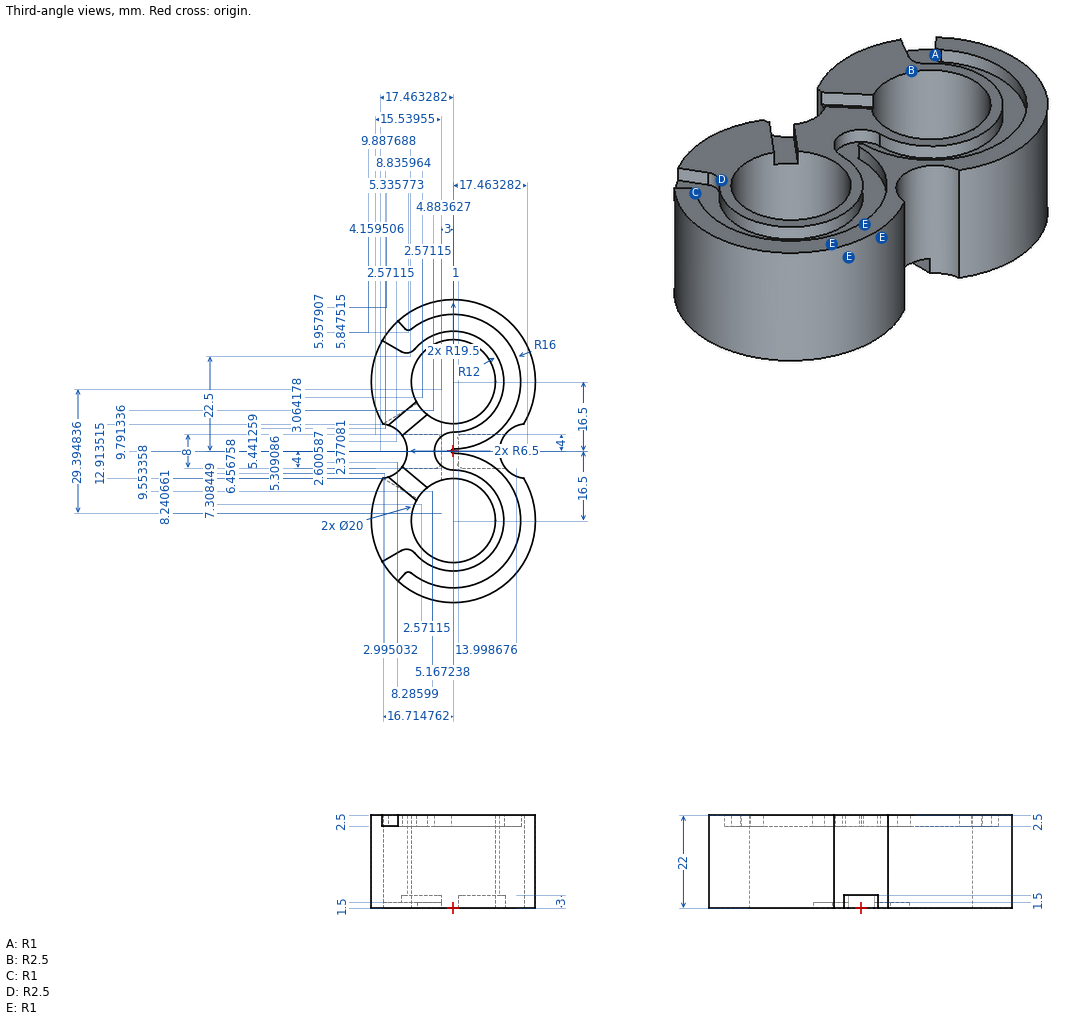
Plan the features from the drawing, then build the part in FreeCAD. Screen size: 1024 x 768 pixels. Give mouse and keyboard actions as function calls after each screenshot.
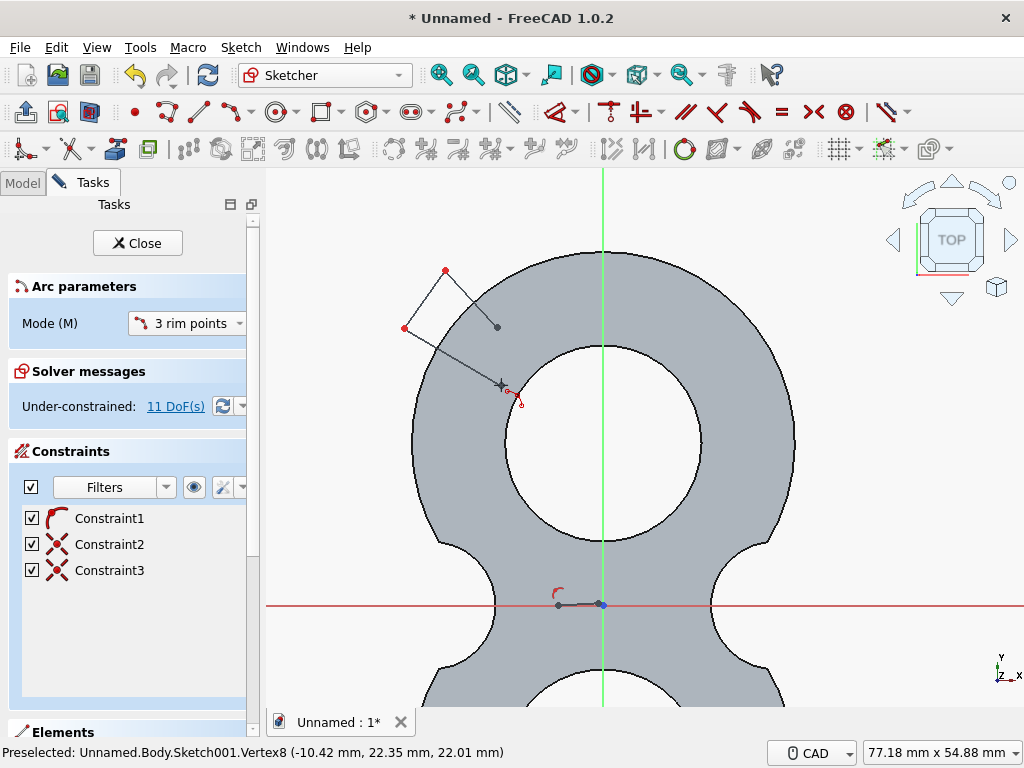
scroll(598, 606, up, 6)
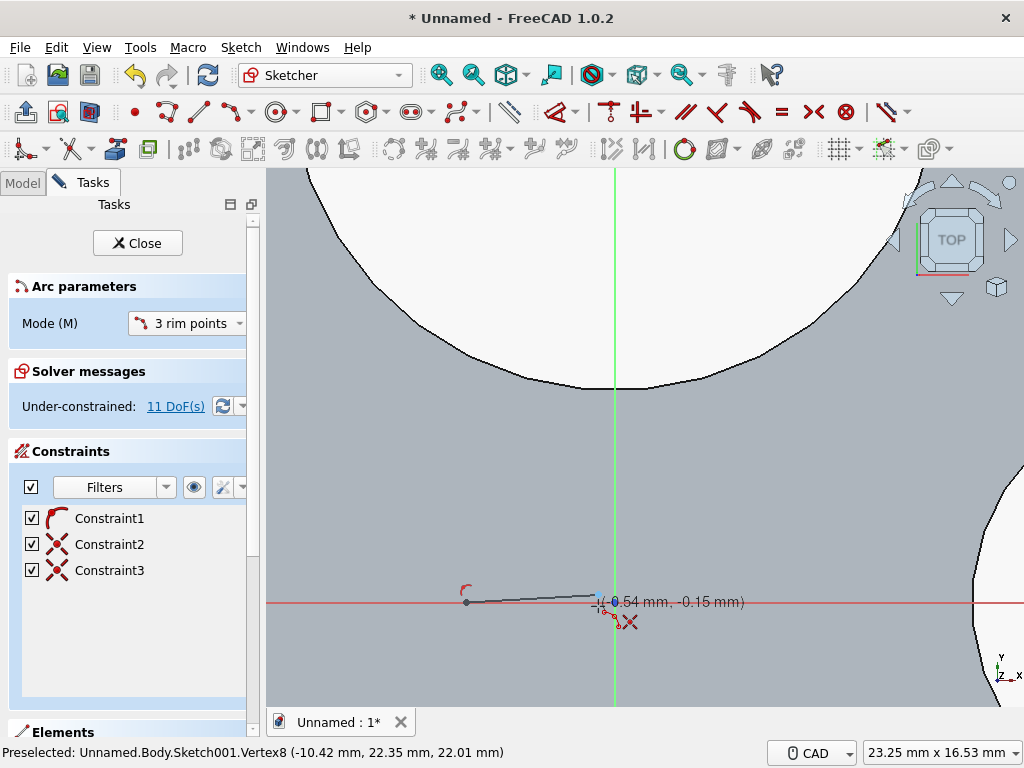
click(598, 595)
click(615, 586)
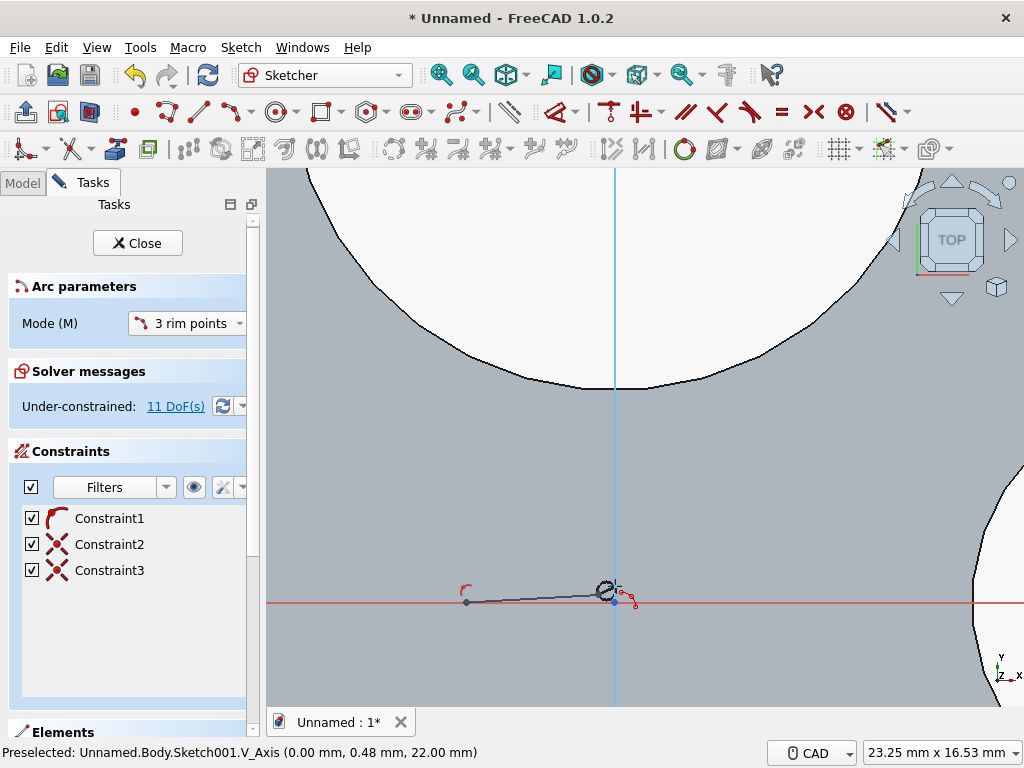
scroll(603, 591, up, 7)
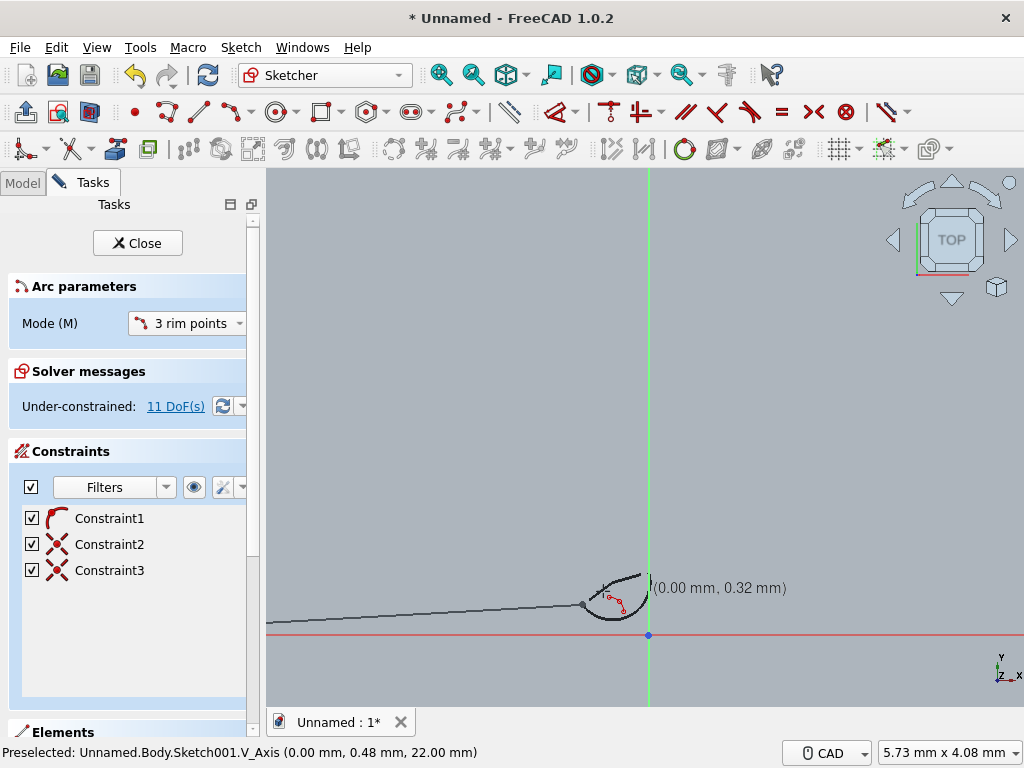
click(602, 589)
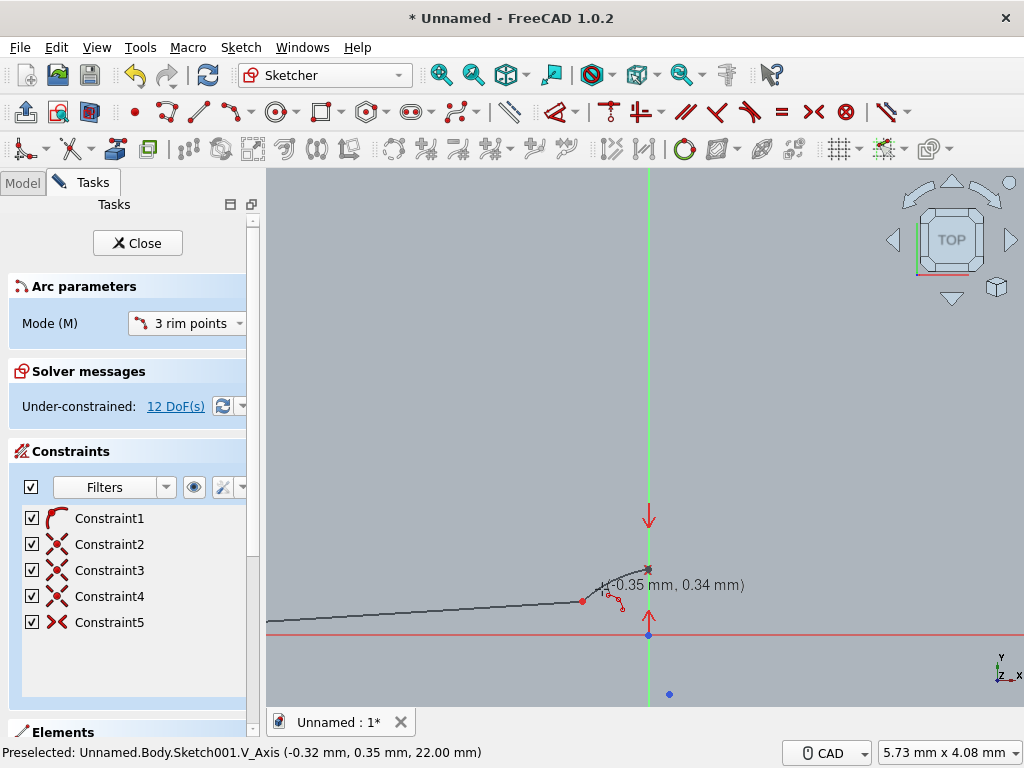
scroll(599, 603, down, 13)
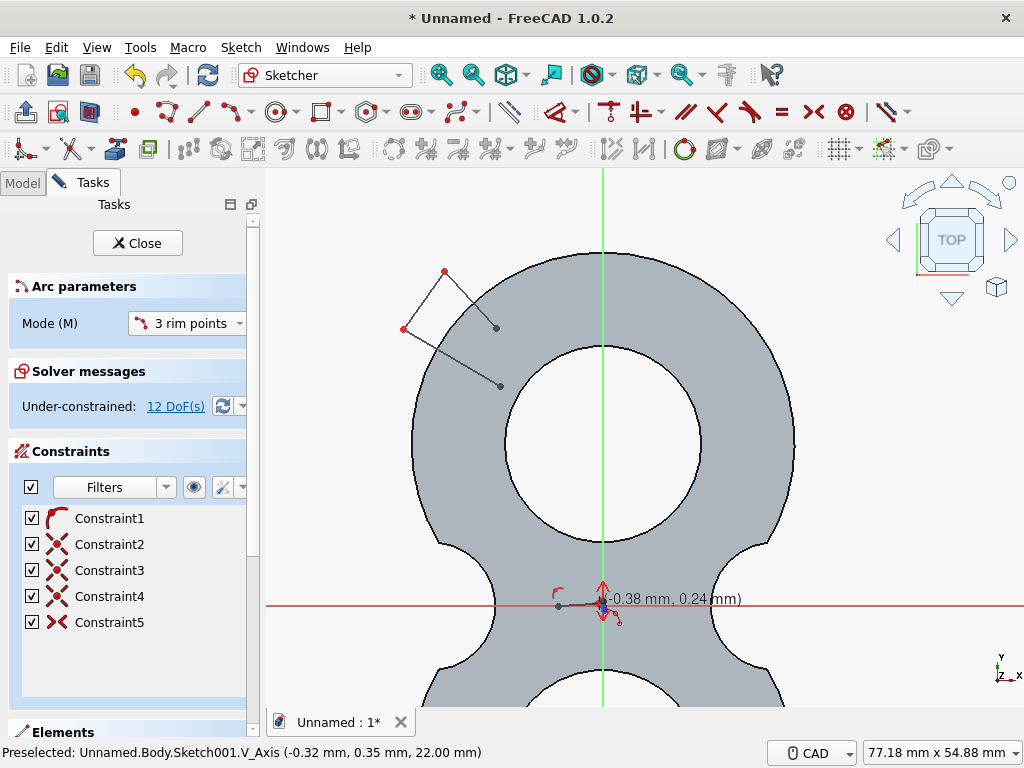
scroll(603, 601, up, 6)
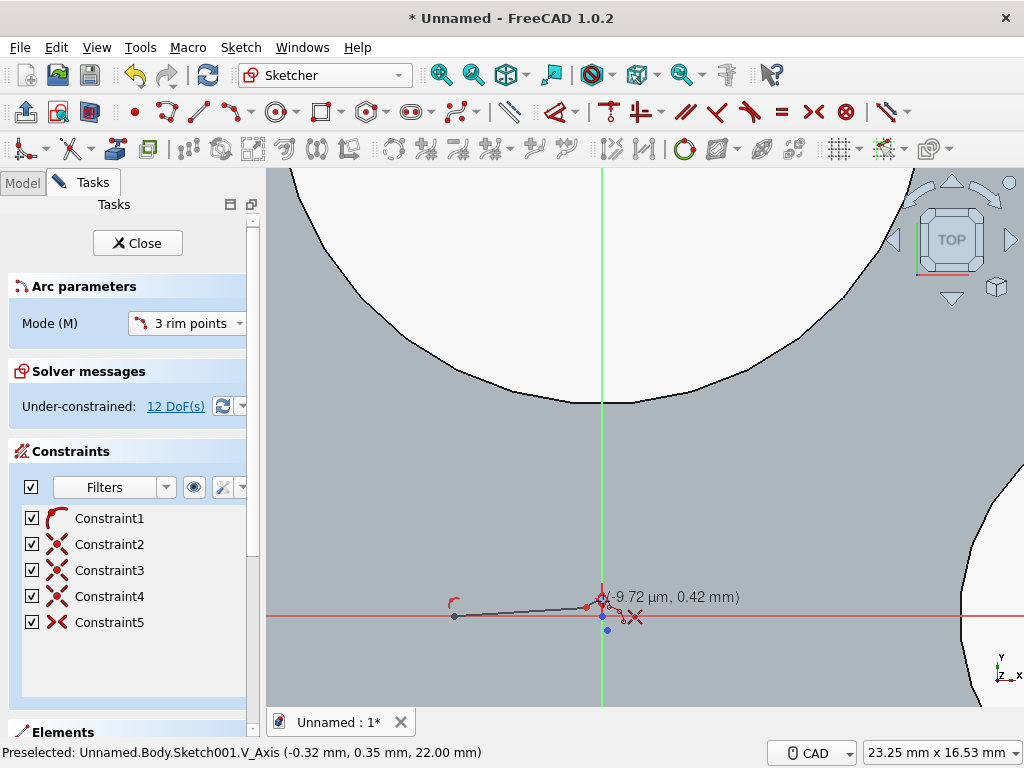
click(602, 600)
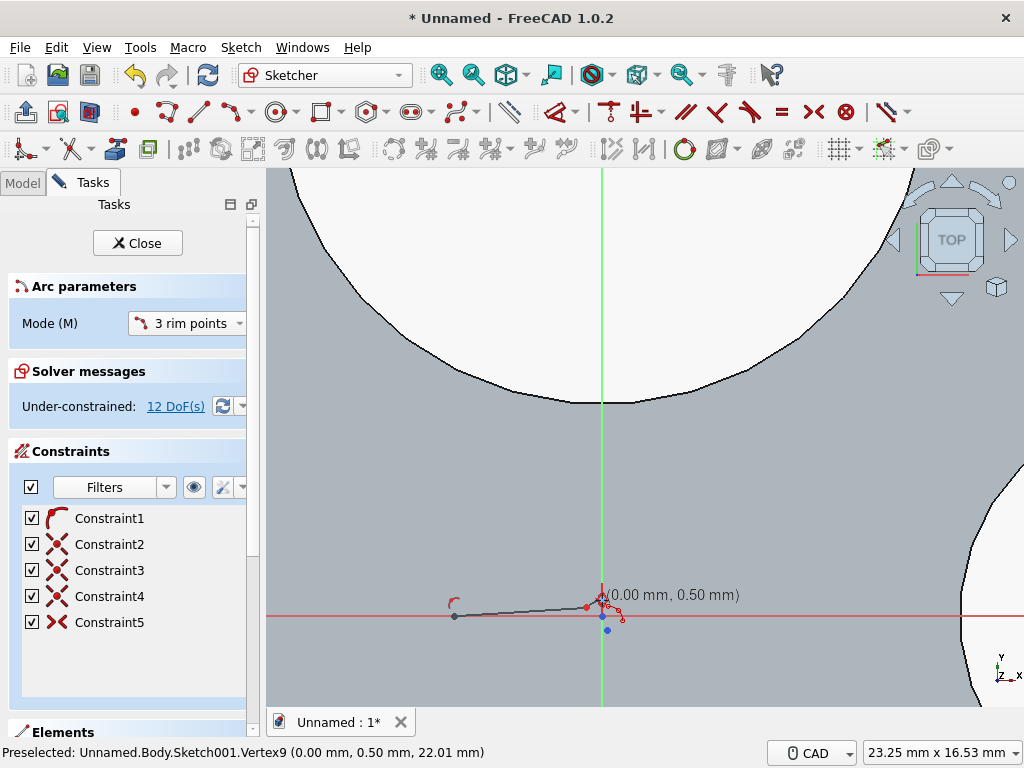
scroll(603, 601, down, 6)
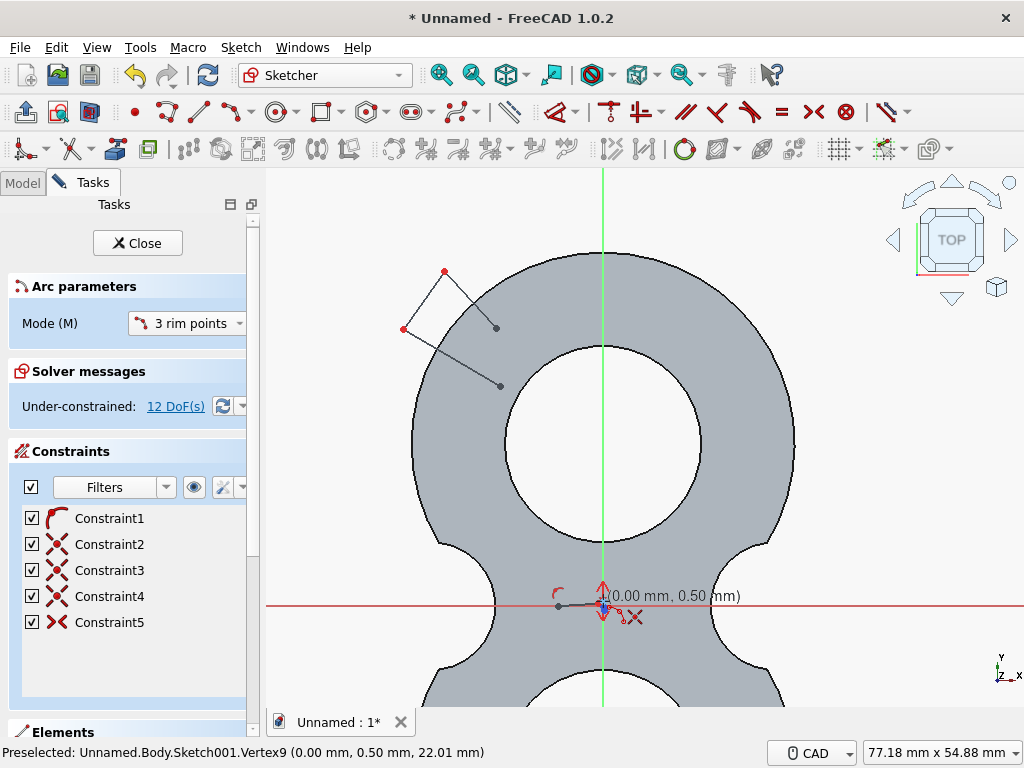
click(497, 329)
click(750, 387)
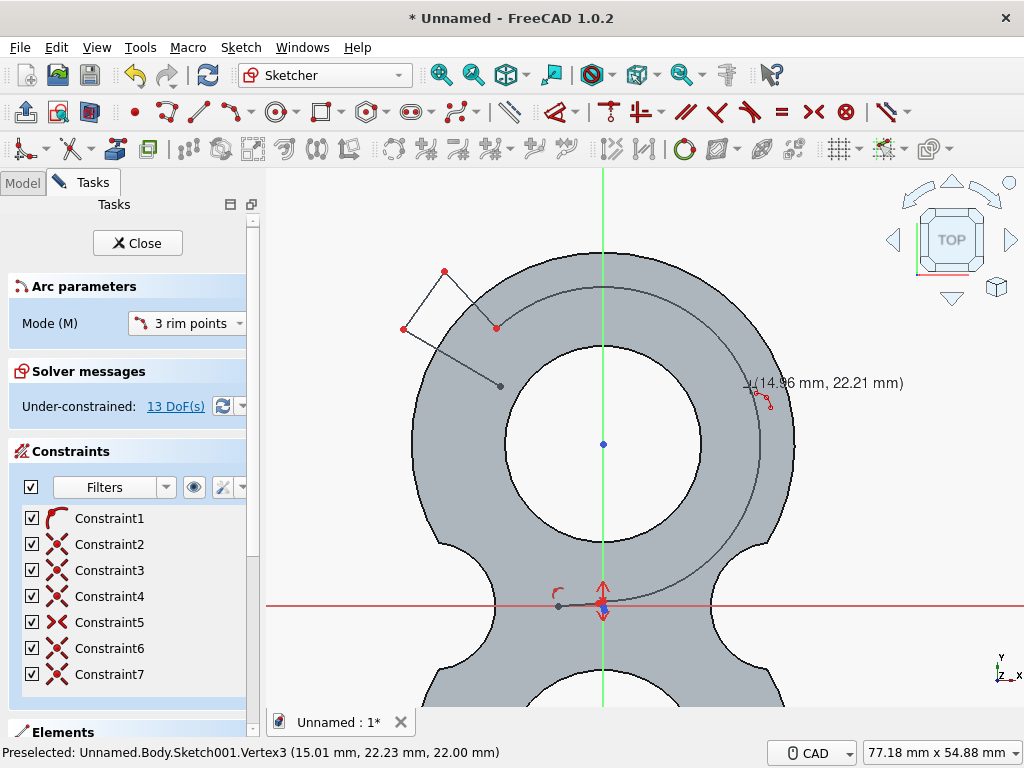
click(501, 387)
click(603, 562)
click(705, 385)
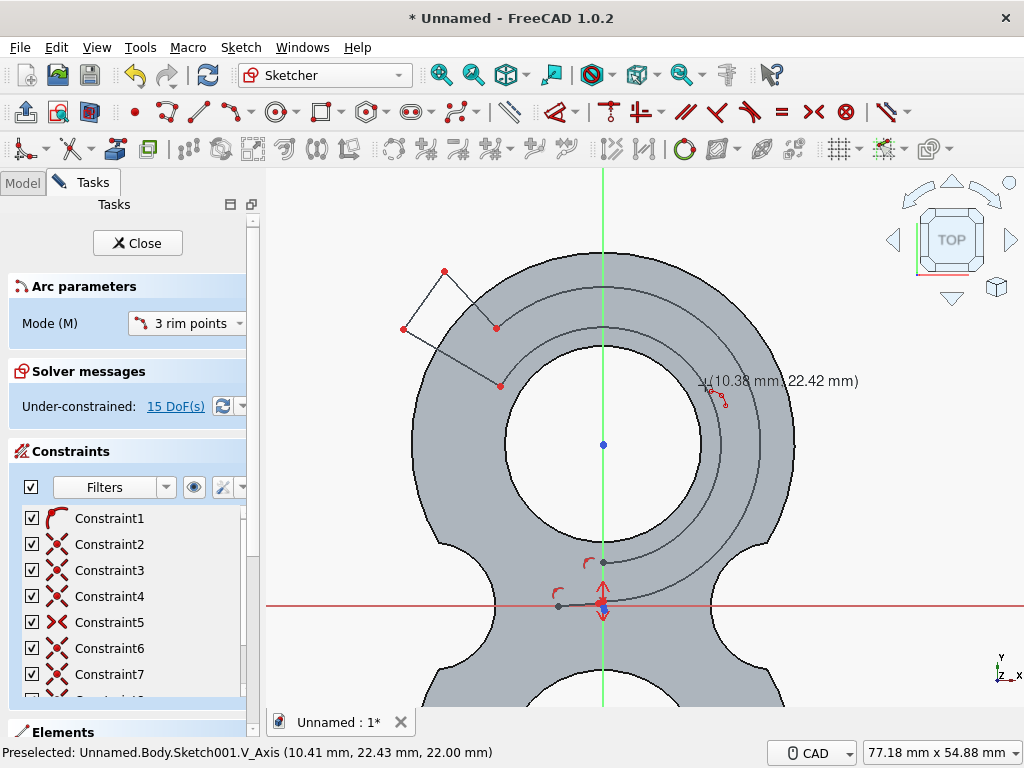
click(603, 563)
click(558, 606)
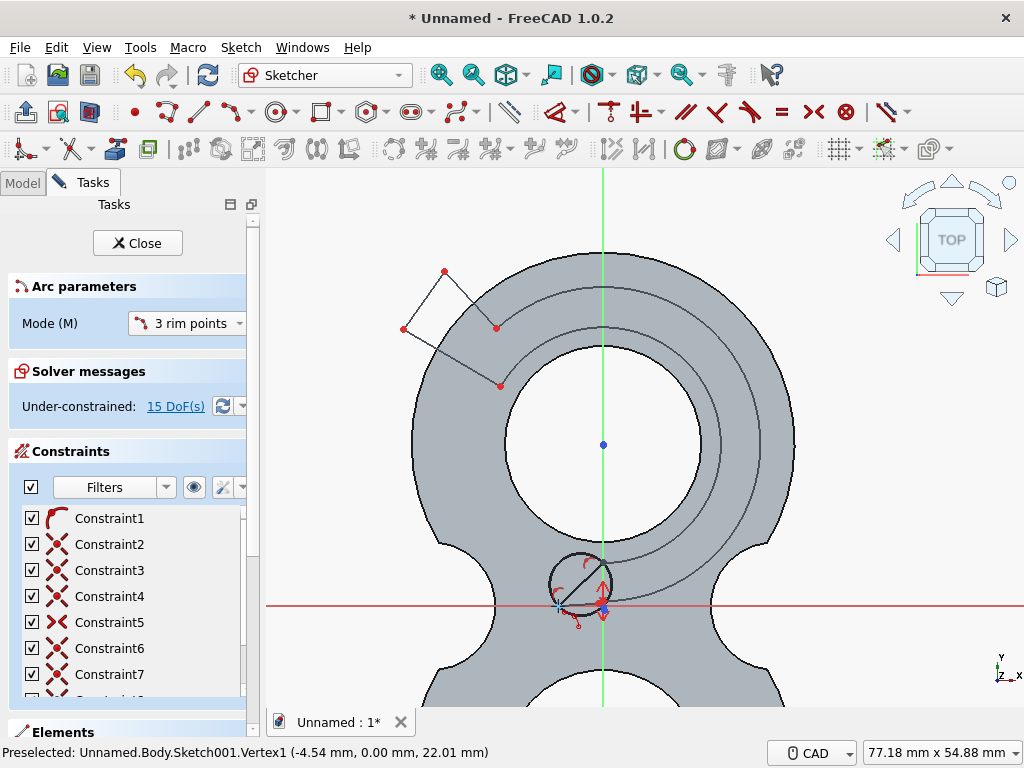
scroll(572, 575, up, 2)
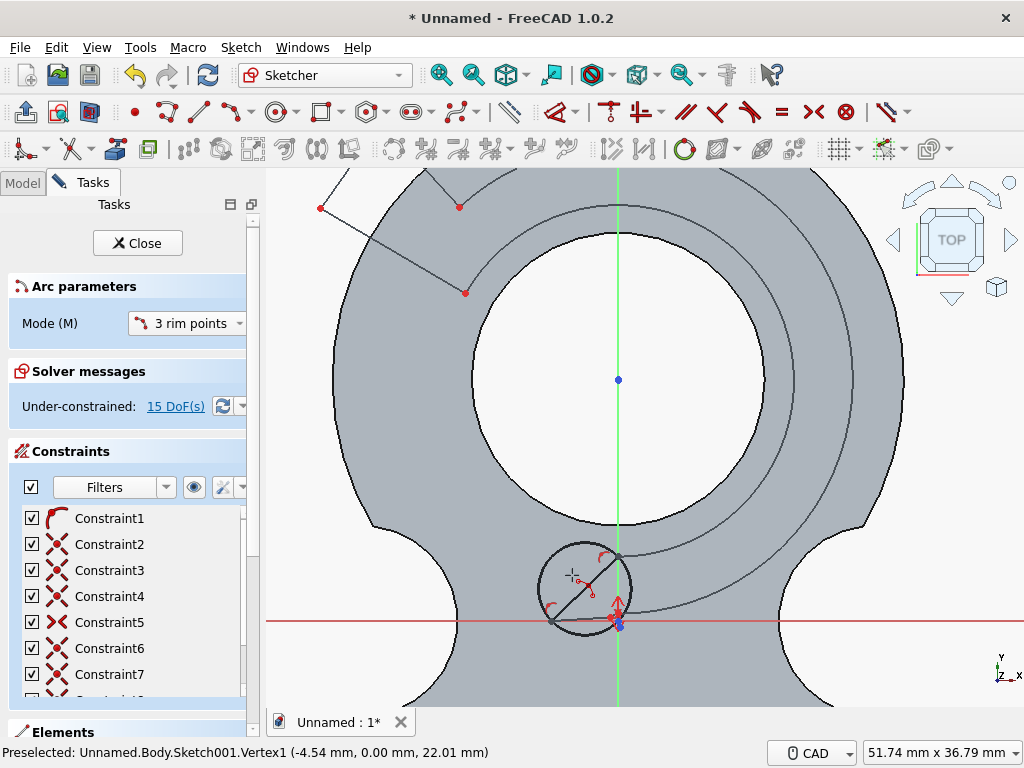
click(572, 574)
key(Escape)